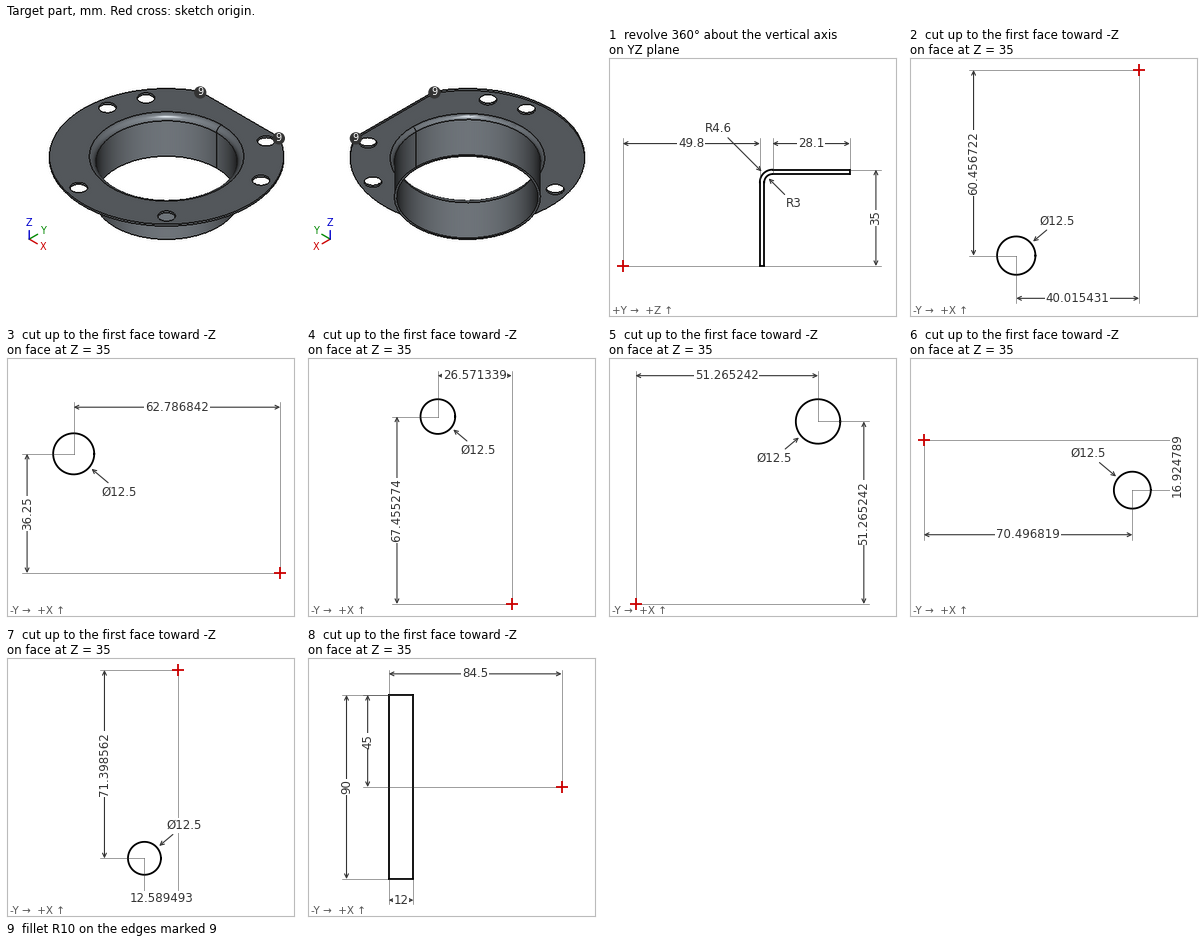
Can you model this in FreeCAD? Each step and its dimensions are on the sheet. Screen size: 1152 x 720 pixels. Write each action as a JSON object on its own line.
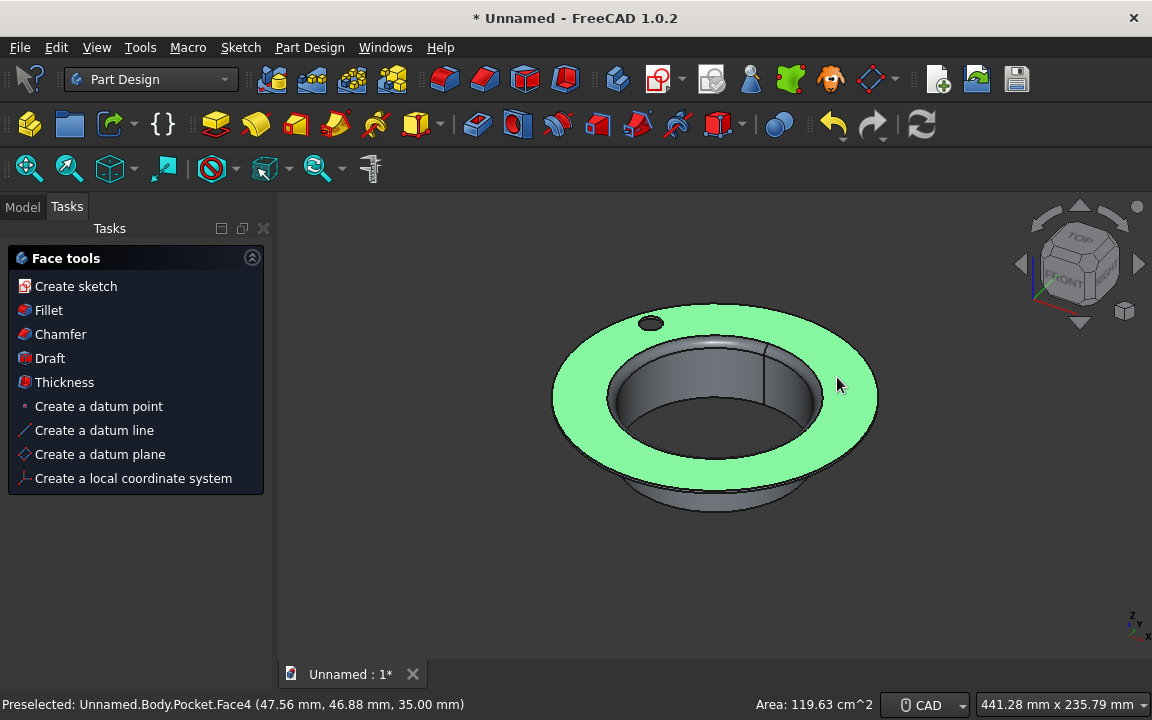
{"action": "left_click", "coordinate": [658, 80]}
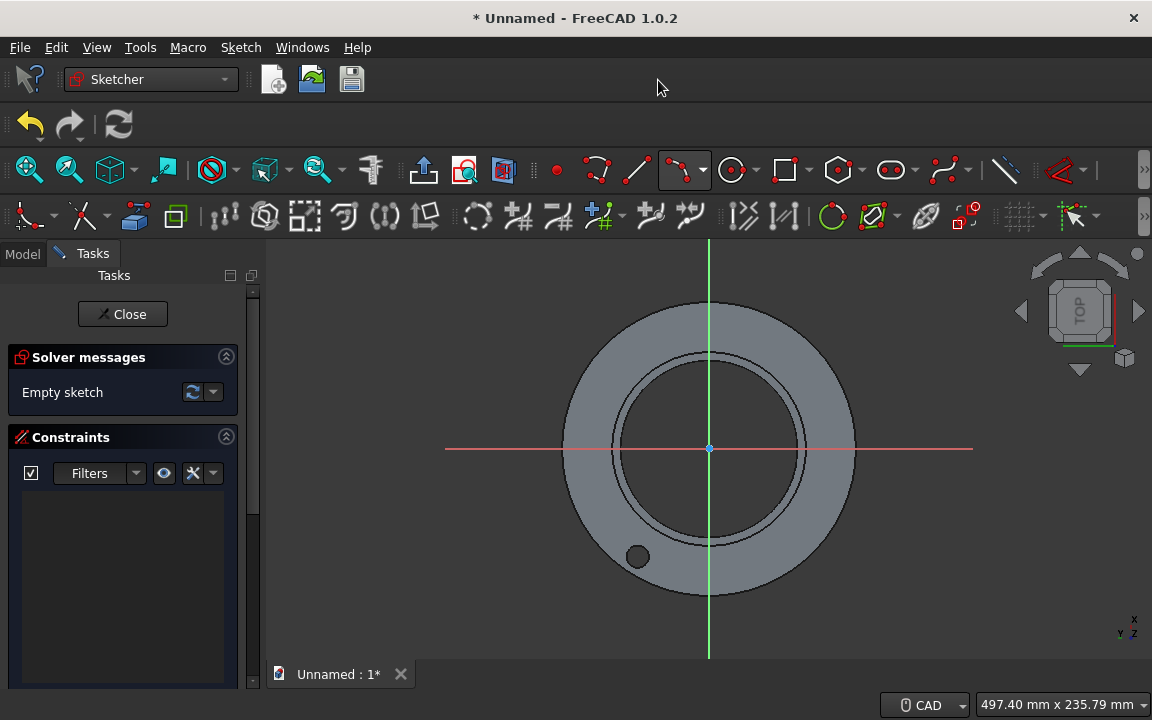
{"action": "scroll", "coordinate": [593, 378], "scroll_direction": "up", "scroll_amount": 12}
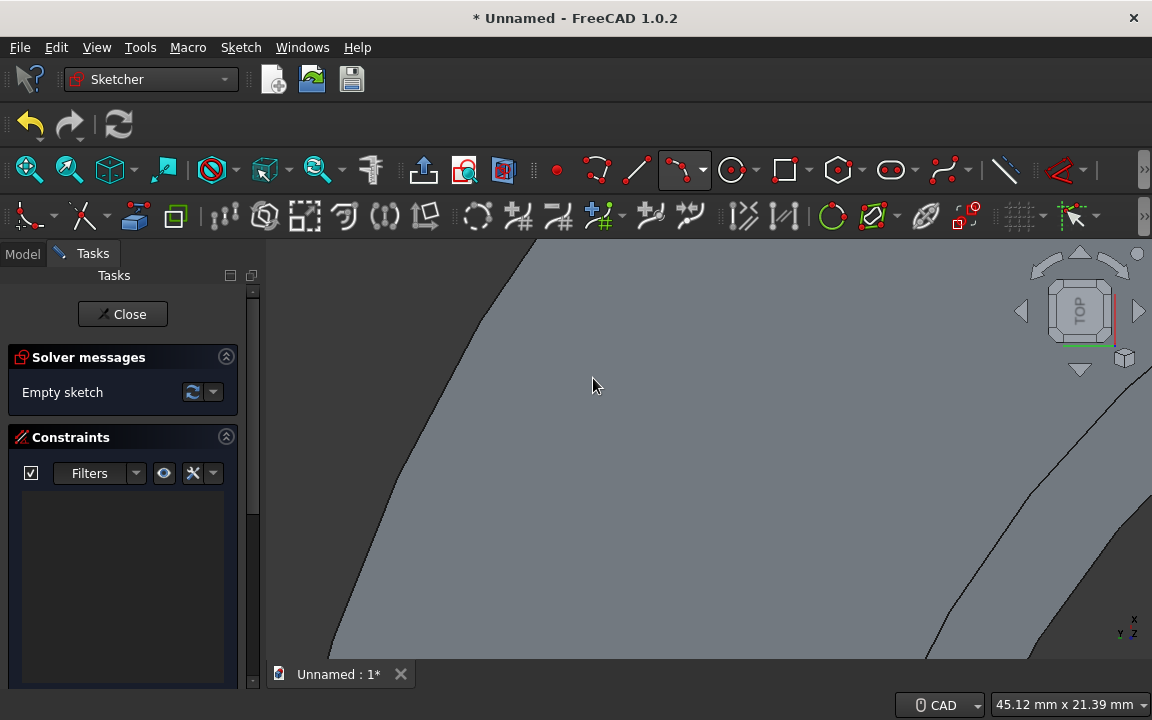
{"action": "key", "text": "g c"}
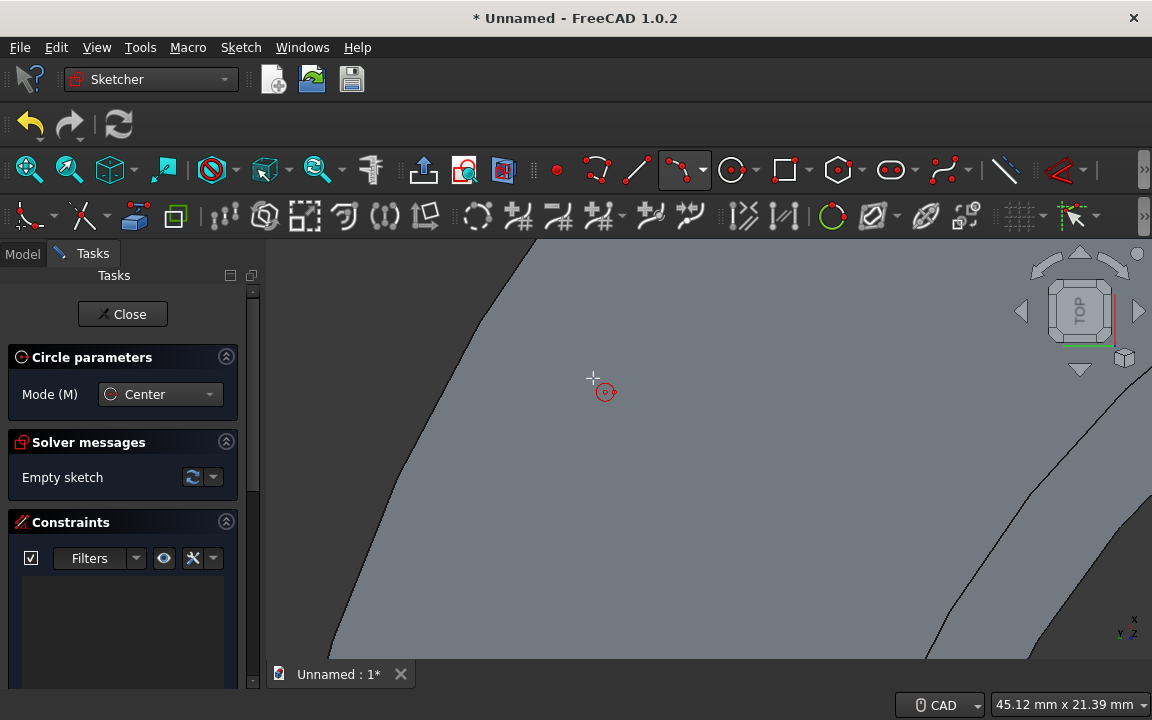
{"action": "left_click", "coordinate": [635, 446]}
{"action": "mouse_move", "coordinate": [722, 359]}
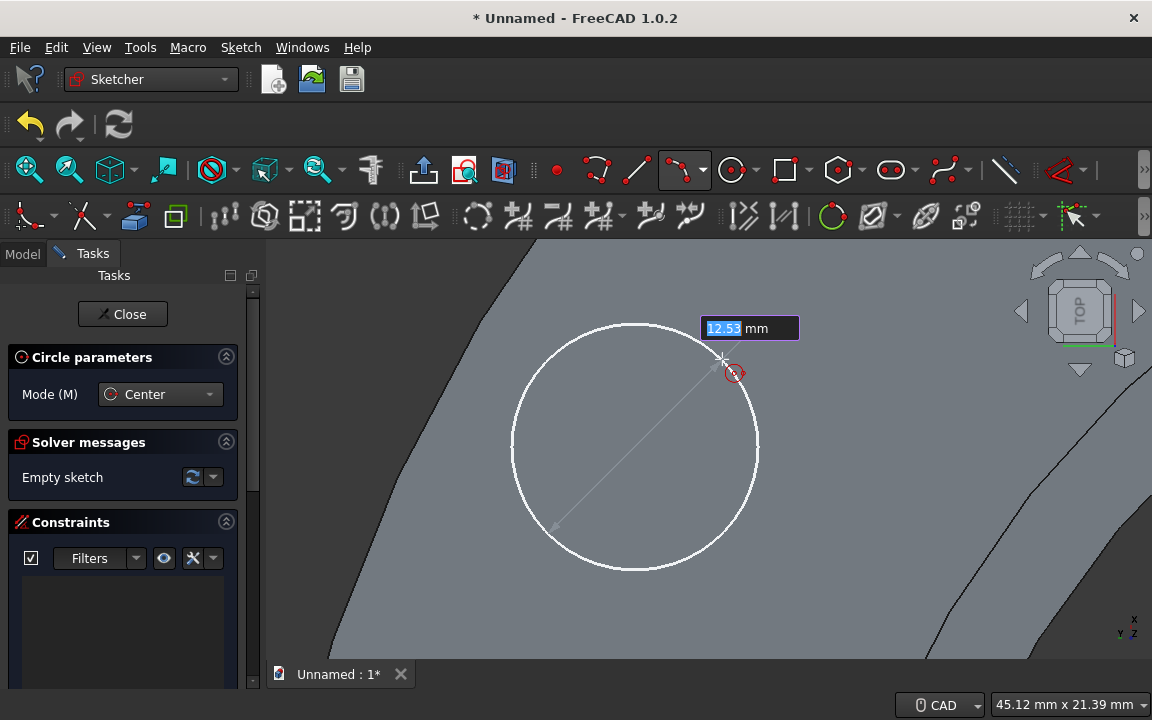
{"action": "type", "text": "12.5"}
{"action": "key", "text": "Return"}
{"action": "key", "text": "Escape"}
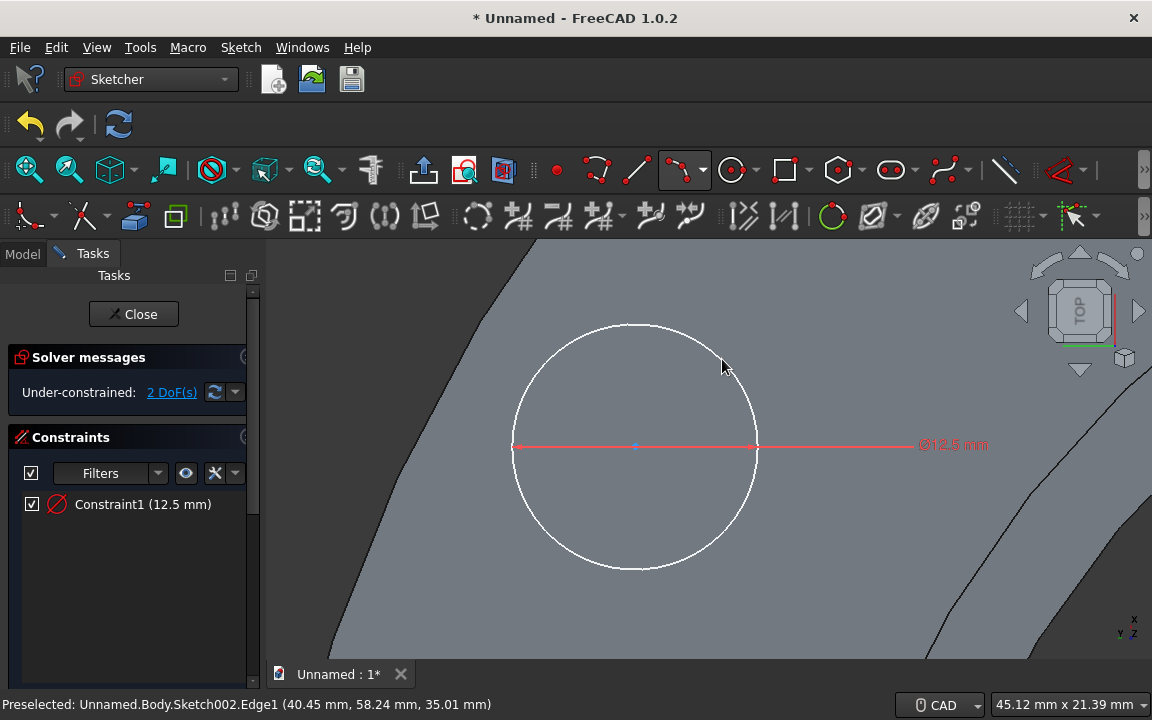
{"action": "left_click", "coordinate": [635, 447]}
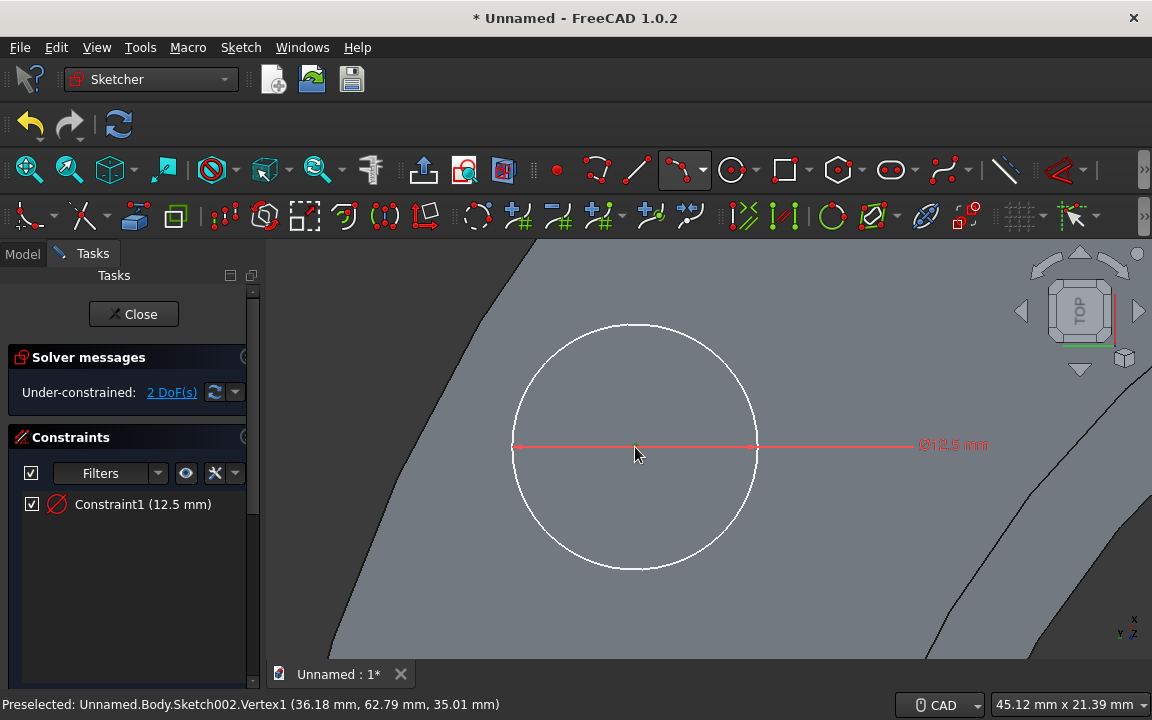
{"action": "left_click", "coordinate": [1086, 170]}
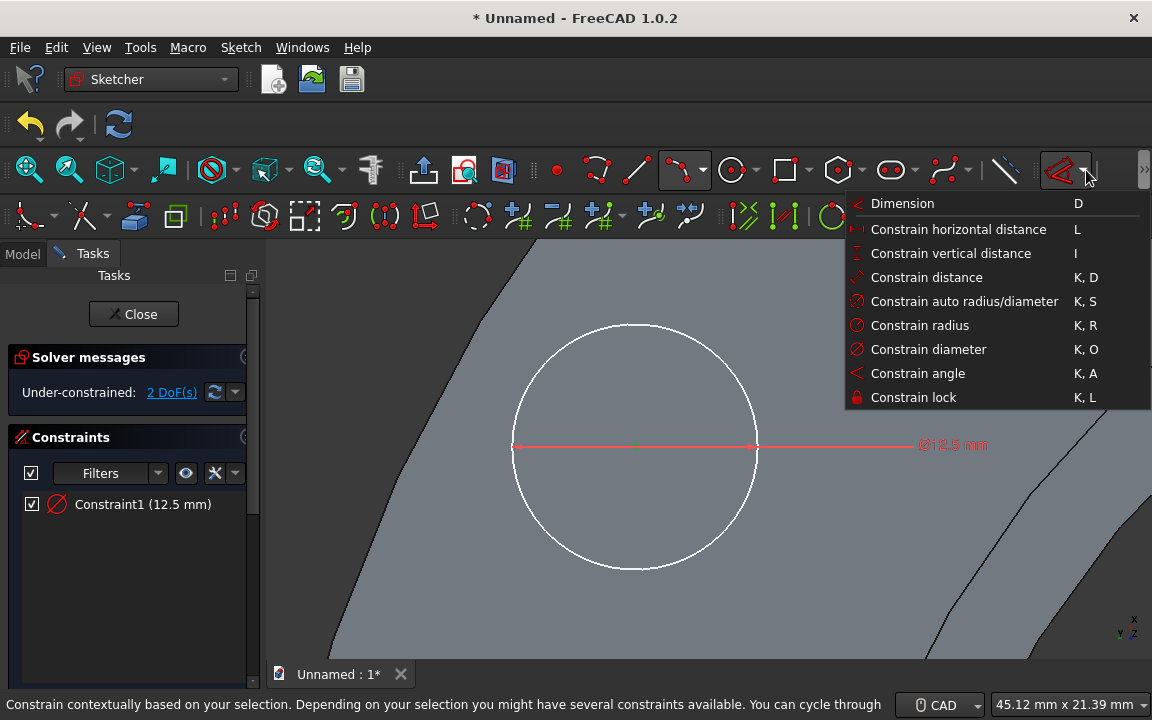
{"action": "left_click", "coordinate": [998, 253]}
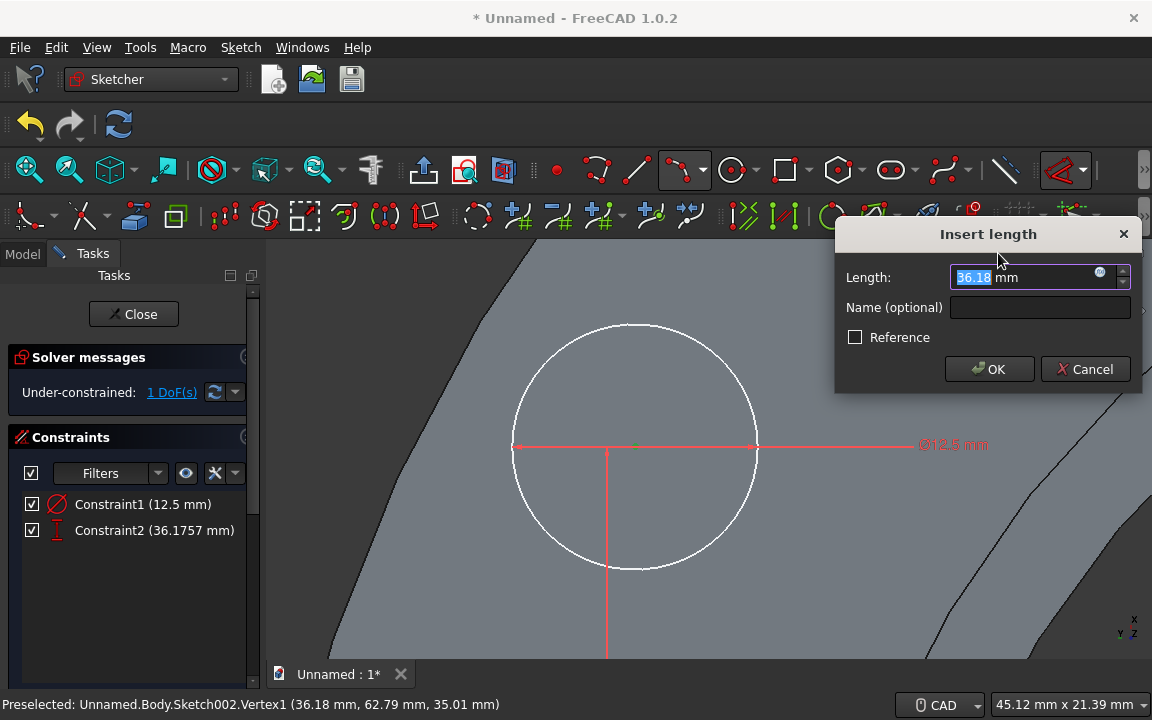
{"action": "type", "text": "36.25"}
{"action": "key", "text": "Return"}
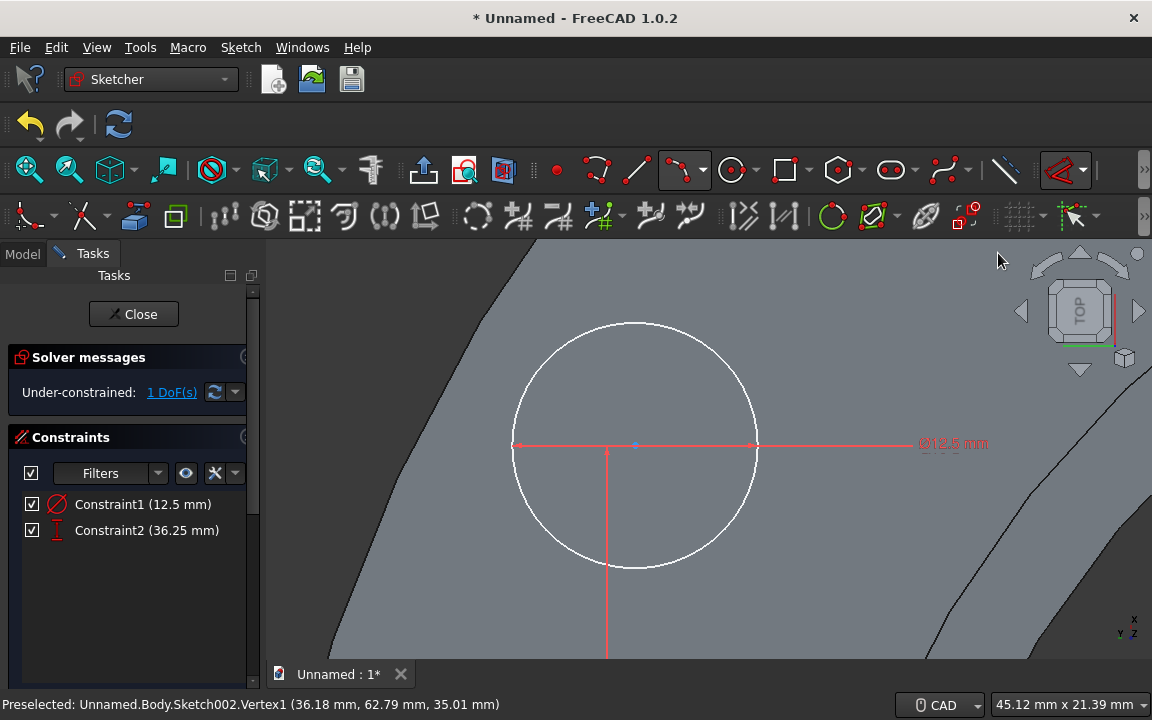
{"action": "left_click", "coordinate": [635, 446]}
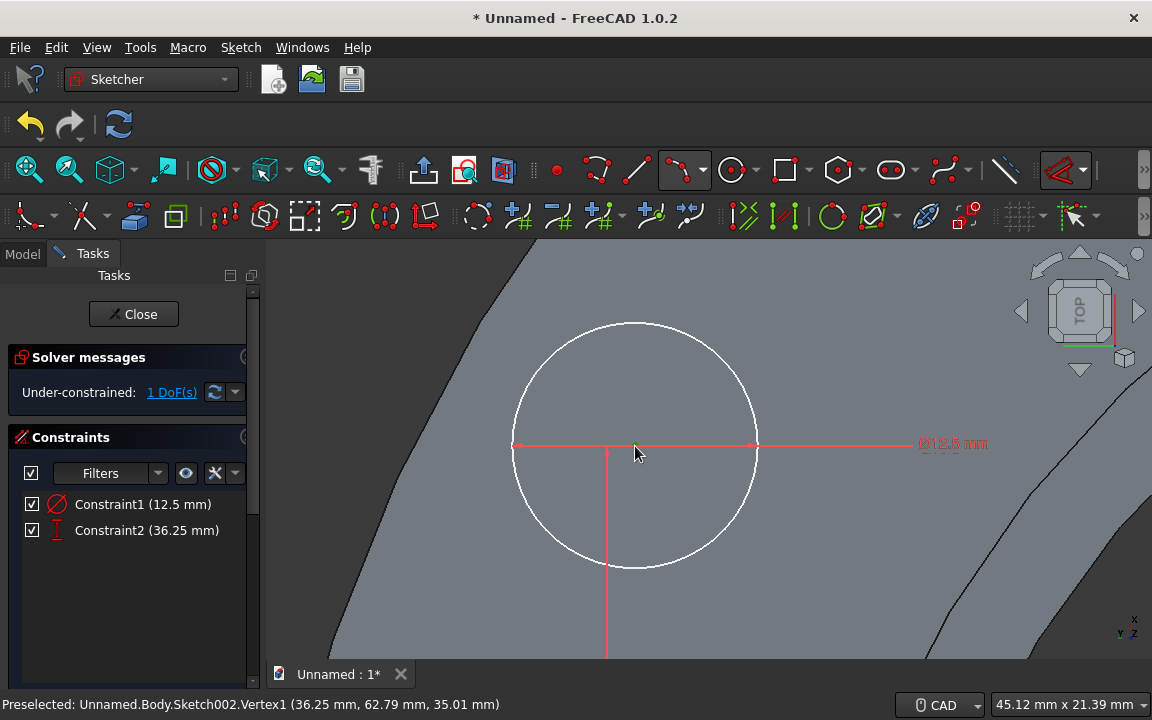
{"action": "key", "text": "l"}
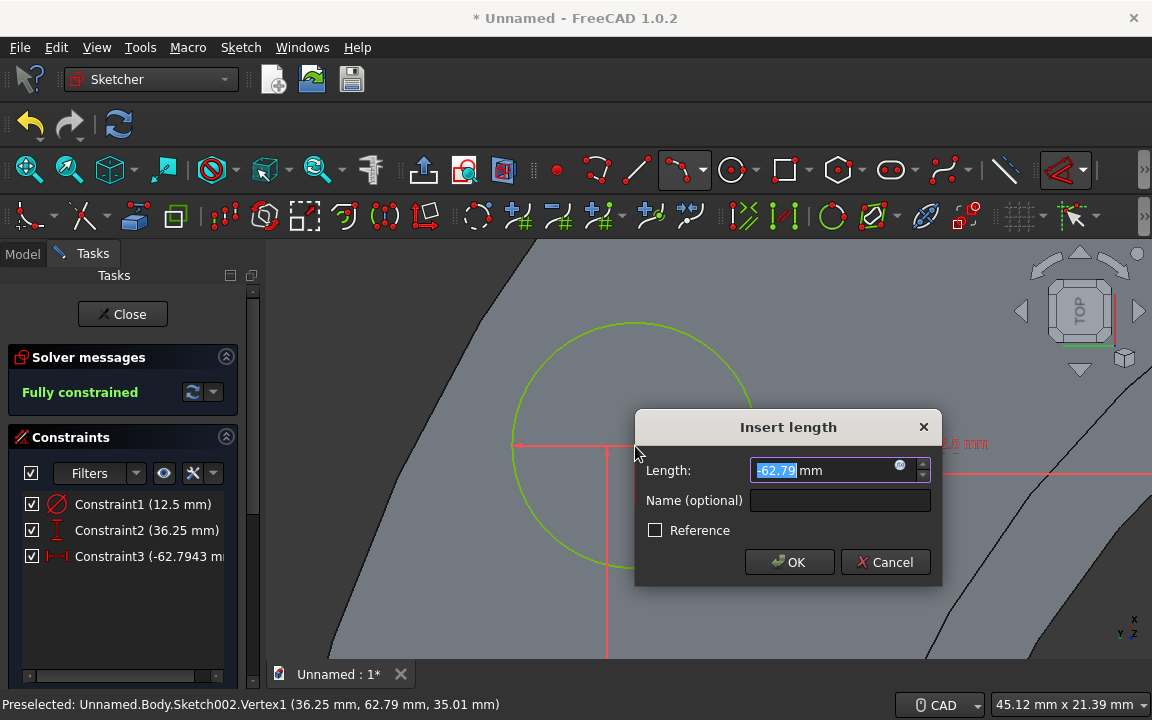
{"action": "type", "text": "-62.786842"}
{"action": "key", "text": "Return"}